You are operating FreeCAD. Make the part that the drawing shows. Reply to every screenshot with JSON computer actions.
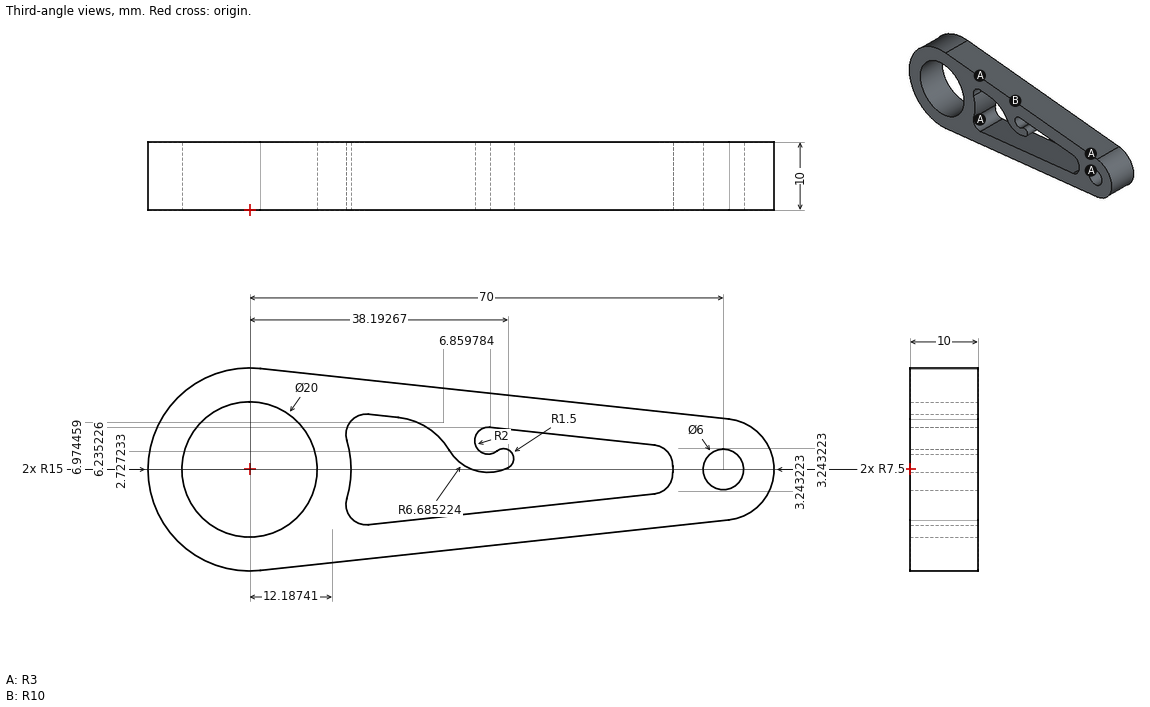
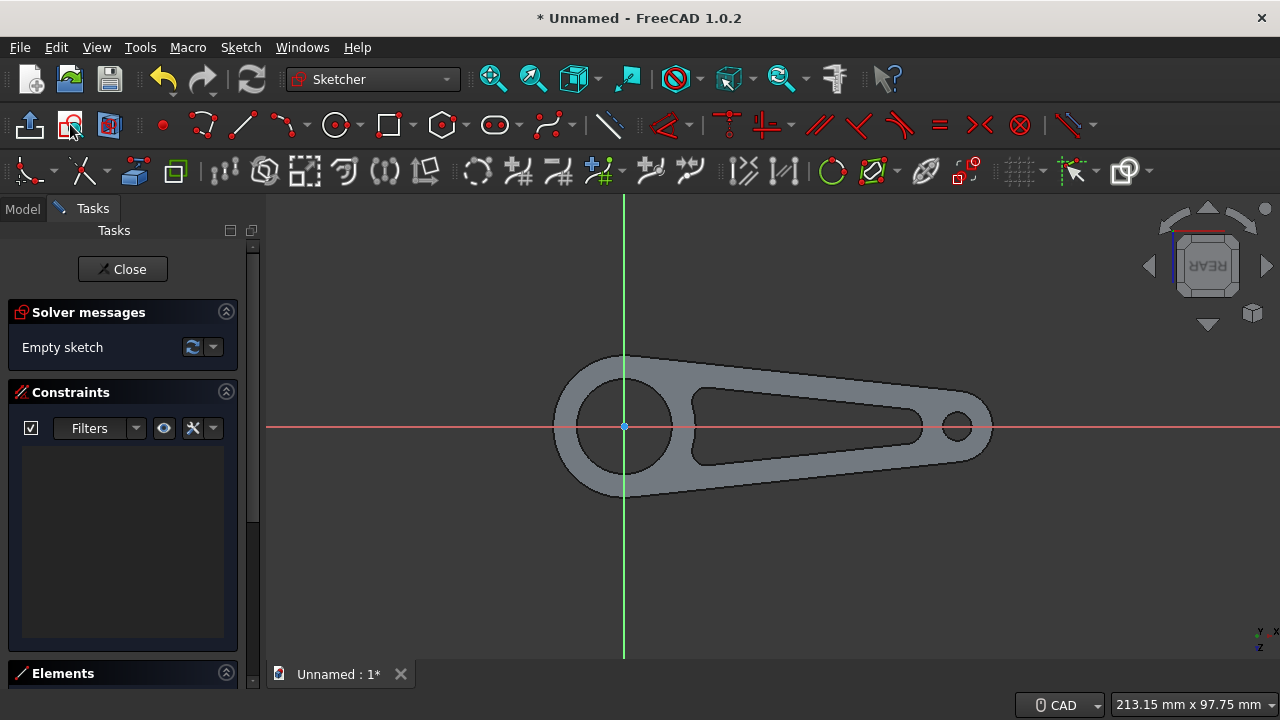
{"action": "scroll", "coordinate": [795, 446], "scroll_direction": "up", "scroll_amount": 11}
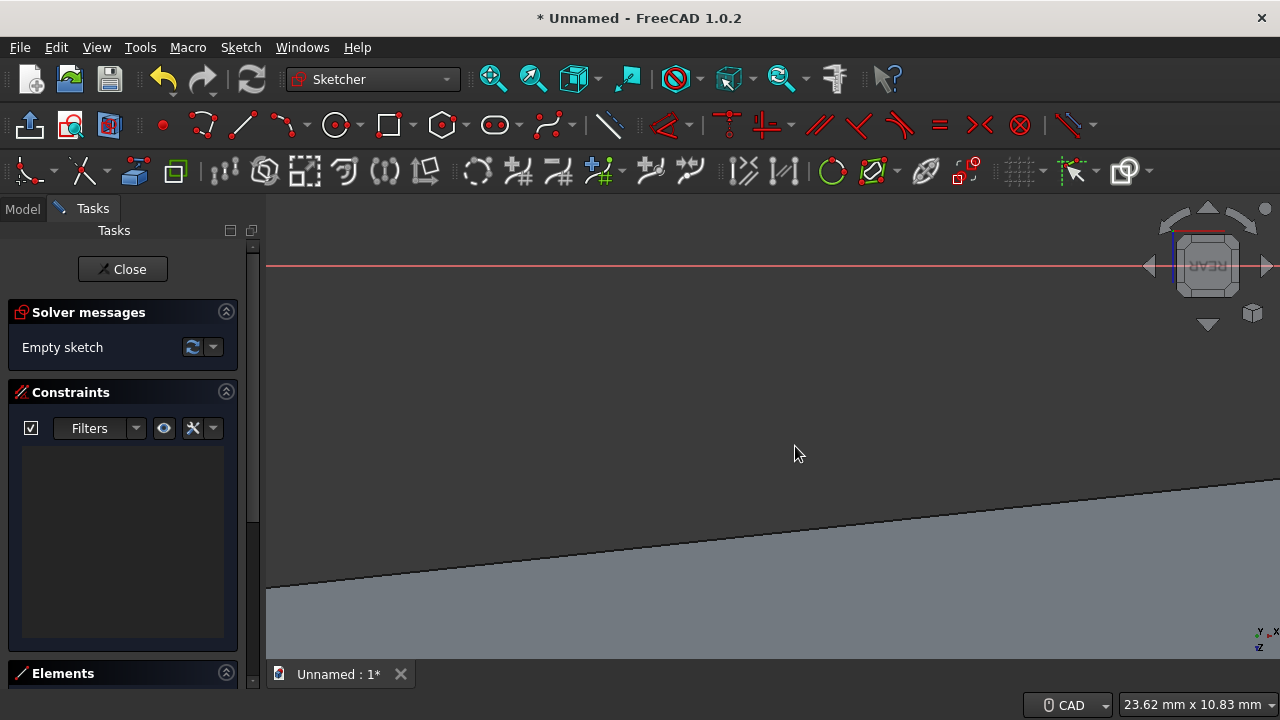
{"action": "left_click", "coordinate": [244, 126]}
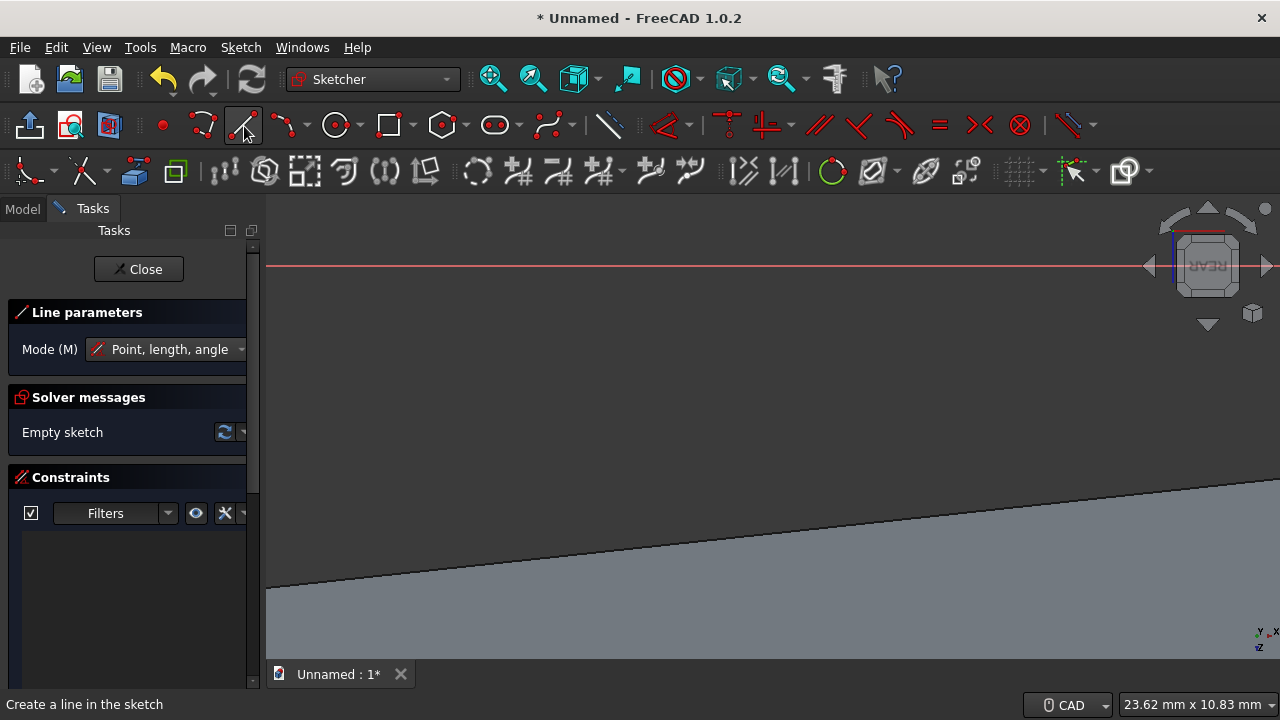
{"action": "left_click", "coordinate": [479, 565]}
{"action": "left_click", "coordinate": [774, 533]}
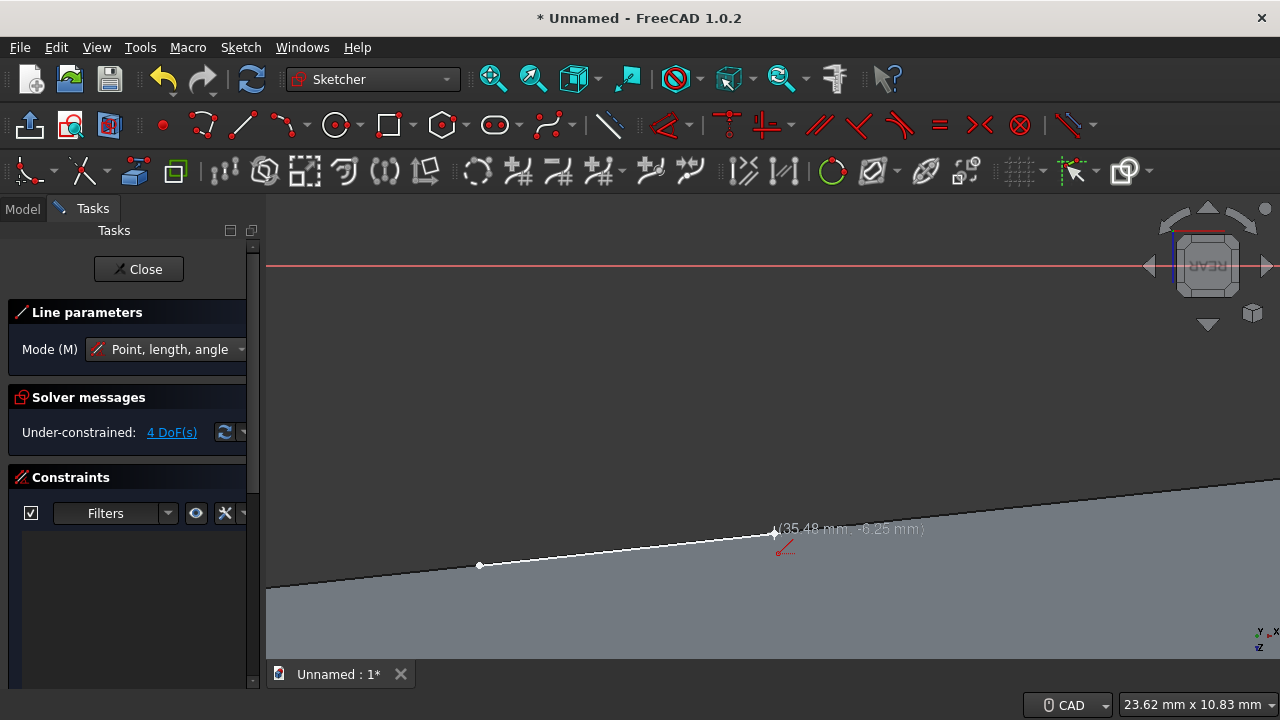
{"action": "key", "text": "g 3 a"}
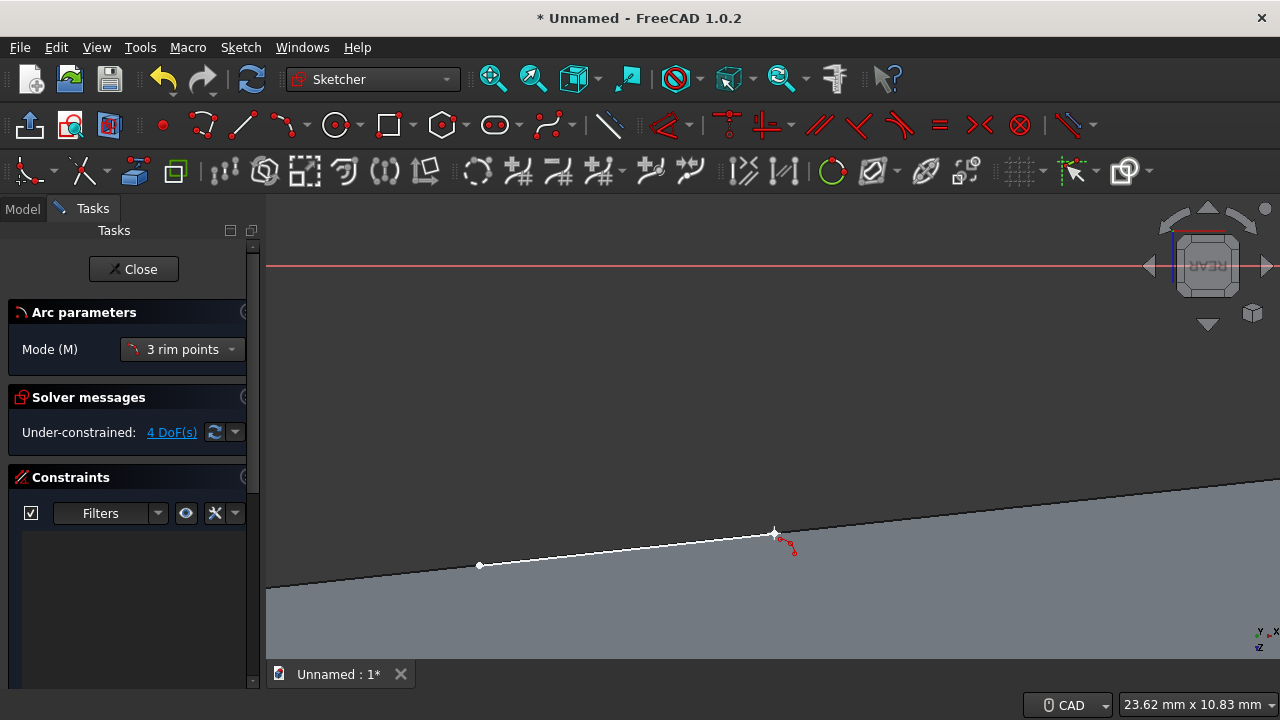
{"action": "left_click", "coordinate": [774, 534]}
{"action": "left_click", "coordinate": [820, 383]}
{"action": "left_click", "coordinate": [682, 423]}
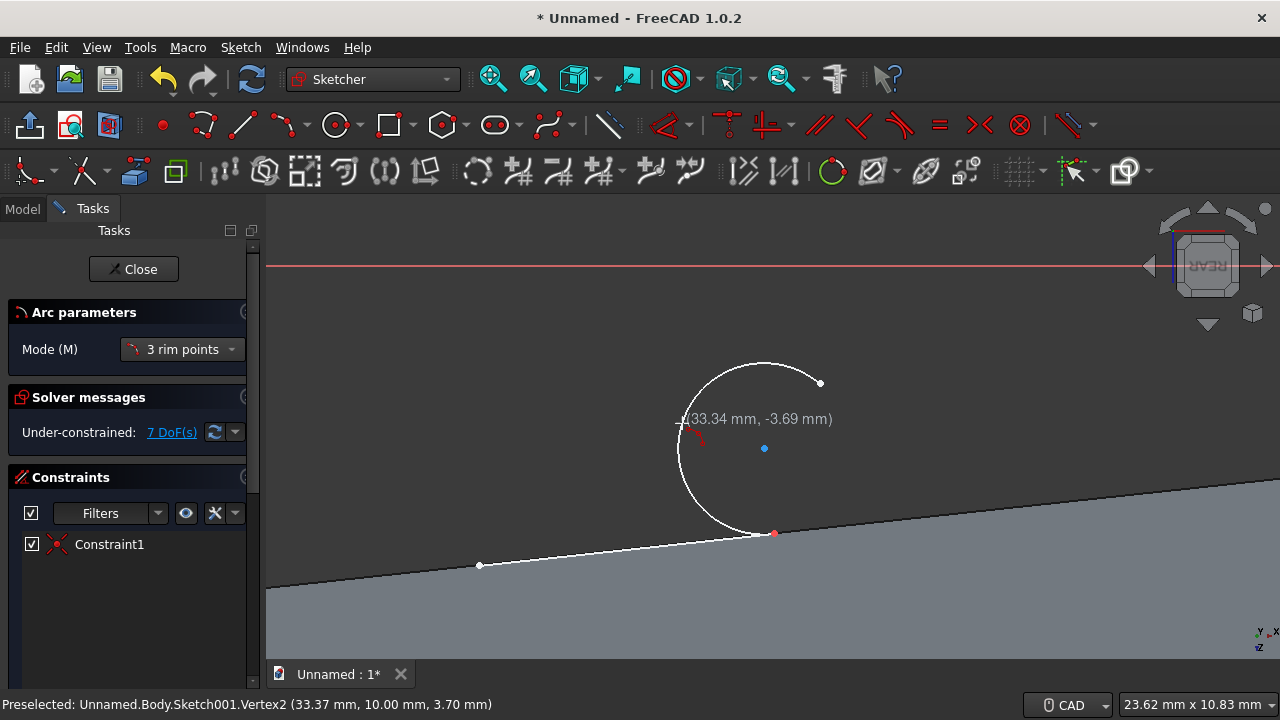
{"action": "left_click", "coordinate": [820, 384]}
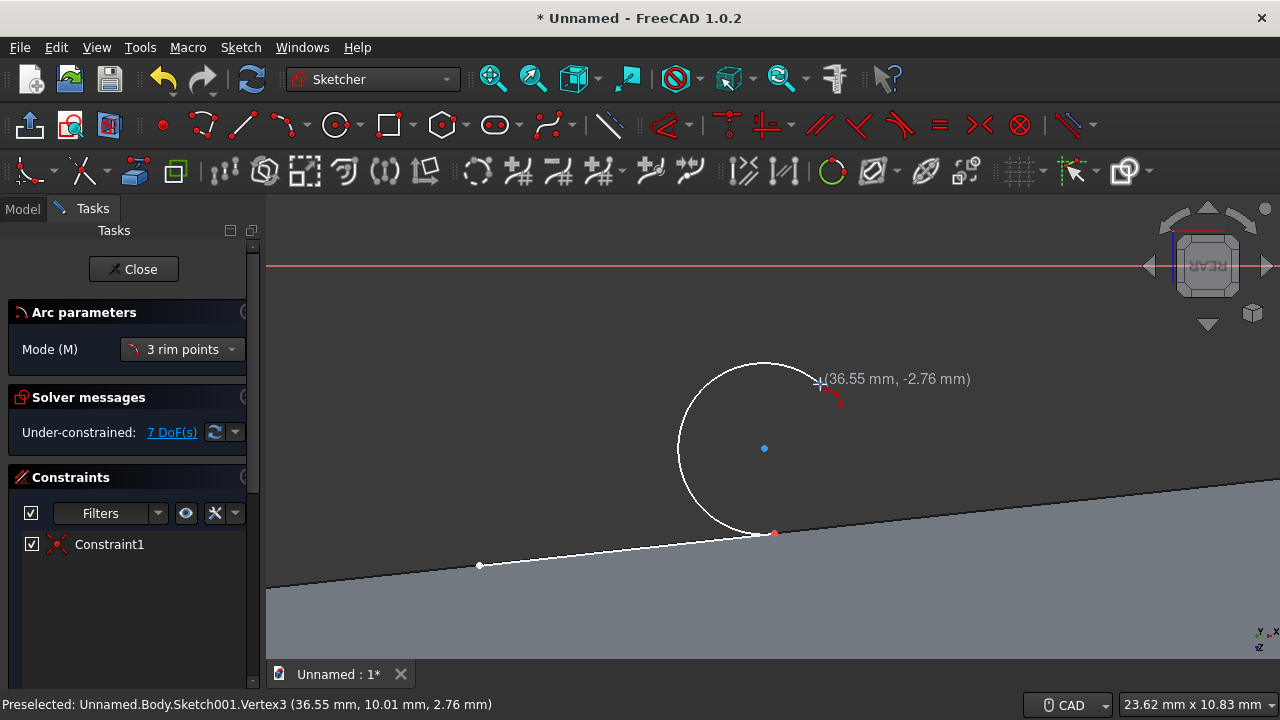
{"action": "scroll", "coordinate": [890, 276], "scroll_direction": "up", "scroll_amount": 3}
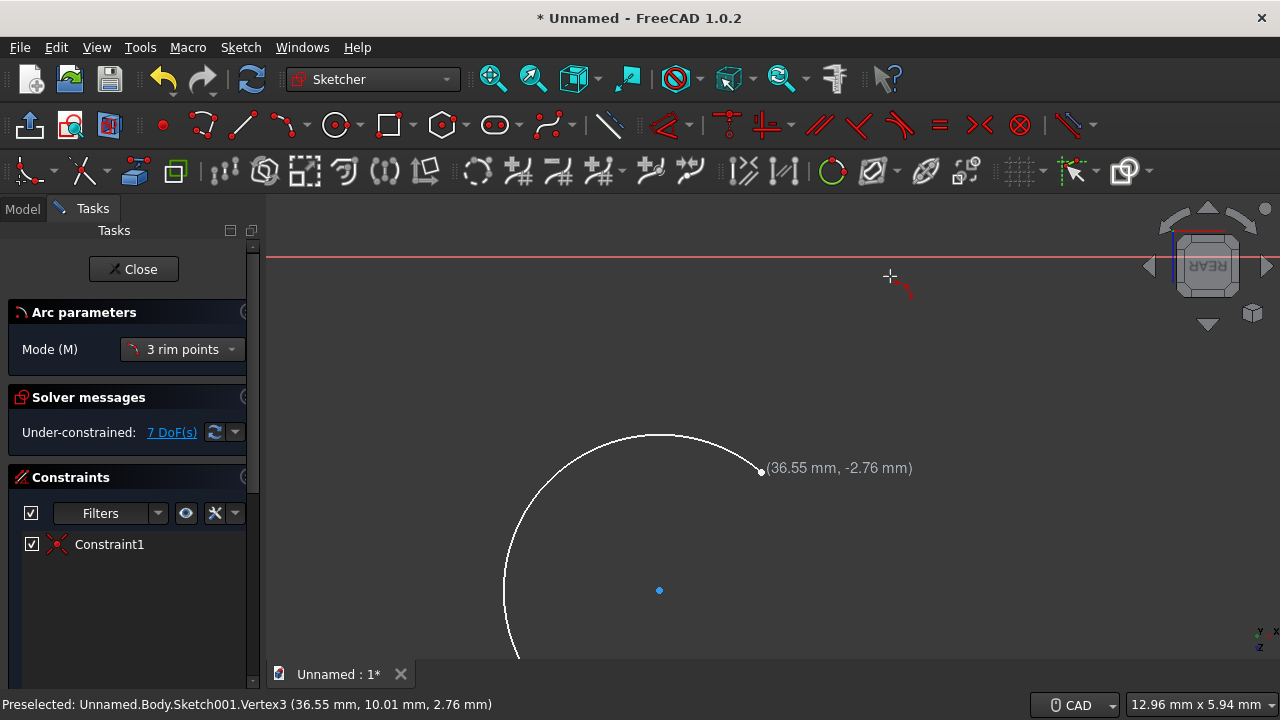
{"action": "left_click", "coordinate": [890, 276]}
{"action": "left_click", "coordinate": [937, 446]}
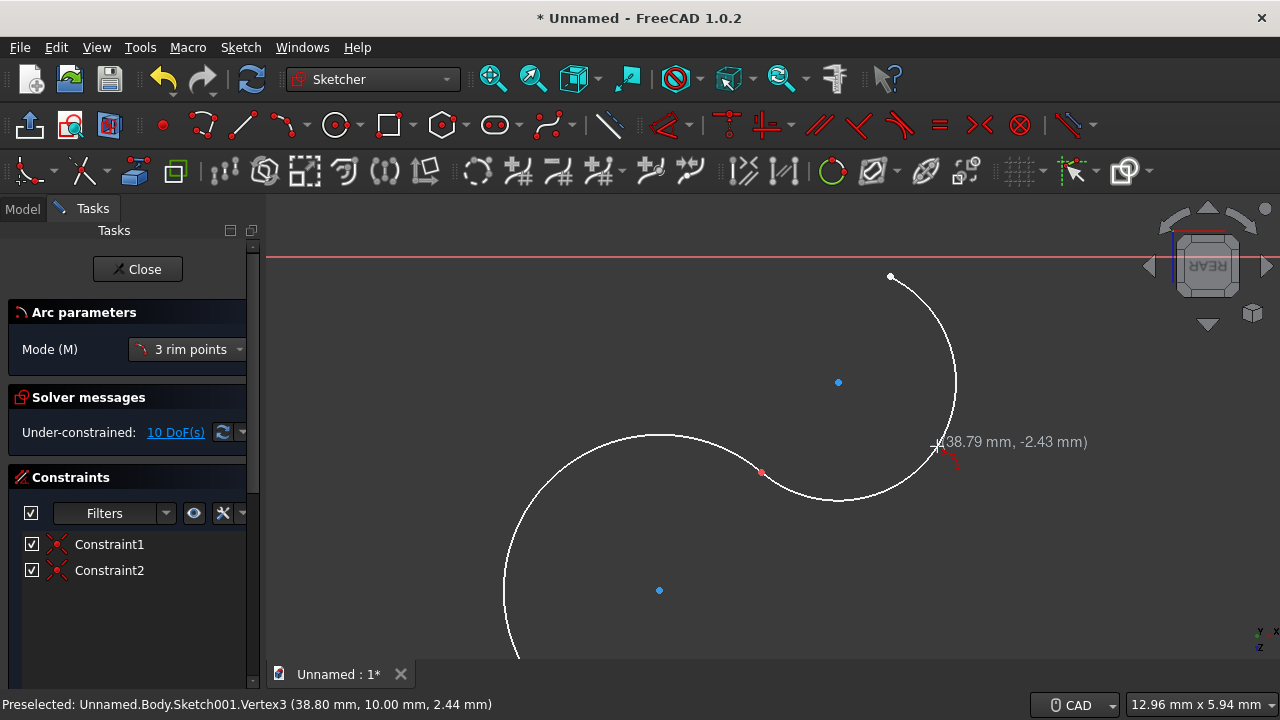
{"action": "left_click", "coordinate": [890, 277]}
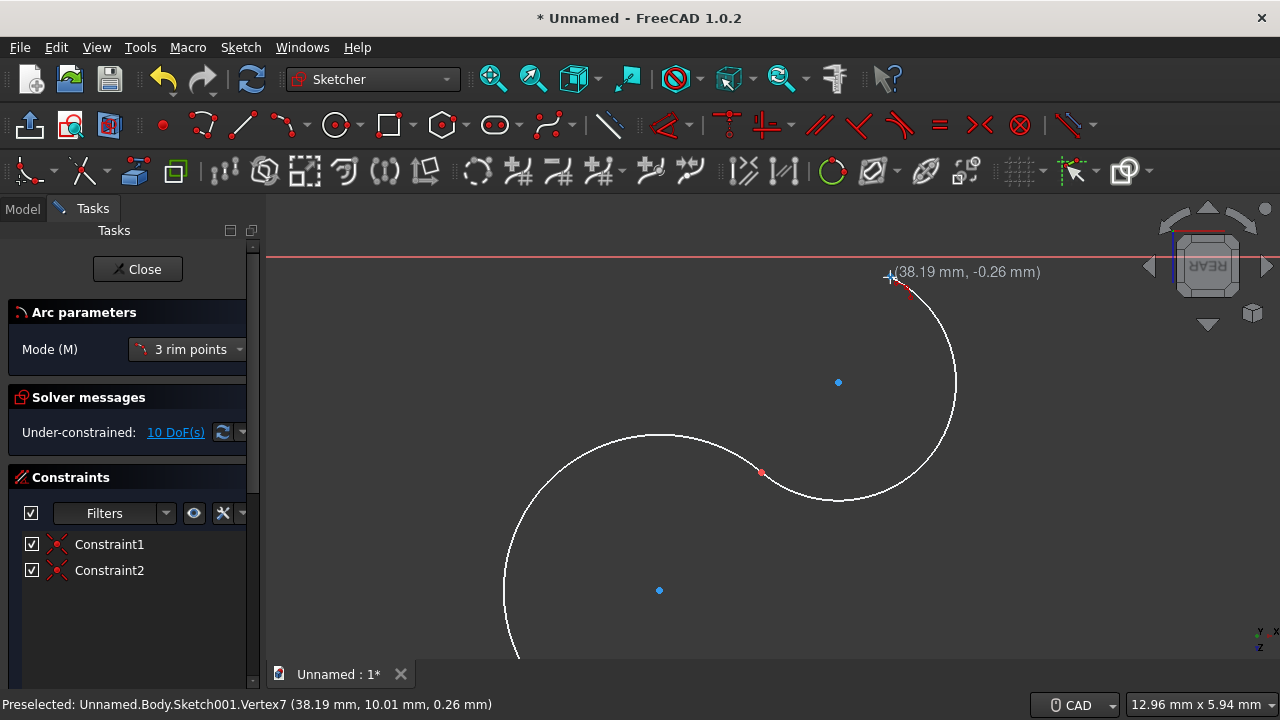
{"action": "scroll", "coordinate": [906, 289], "scroll_direction": "down", "scroll_amount": 3}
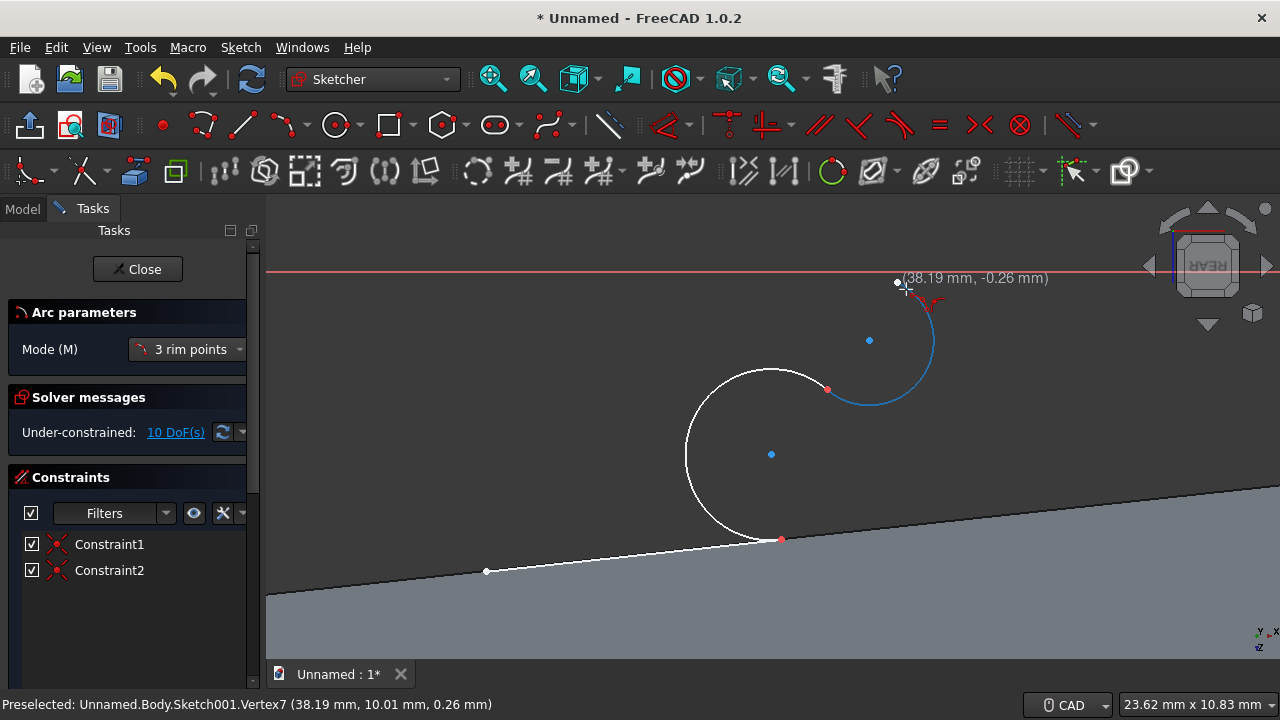
{"action": "left_click", "coordinate": [486, 572]}
{"action": "left_click", "coordinate": [607, 305]}
{"action": "key", "text": "Escape"}